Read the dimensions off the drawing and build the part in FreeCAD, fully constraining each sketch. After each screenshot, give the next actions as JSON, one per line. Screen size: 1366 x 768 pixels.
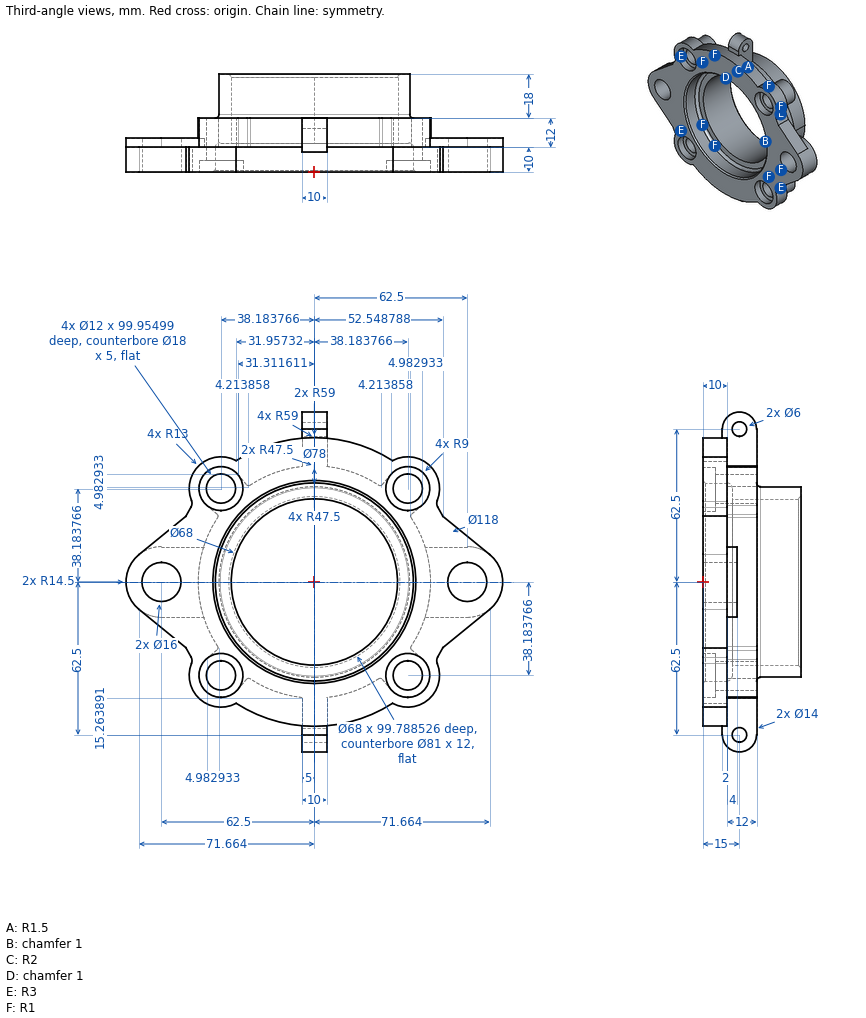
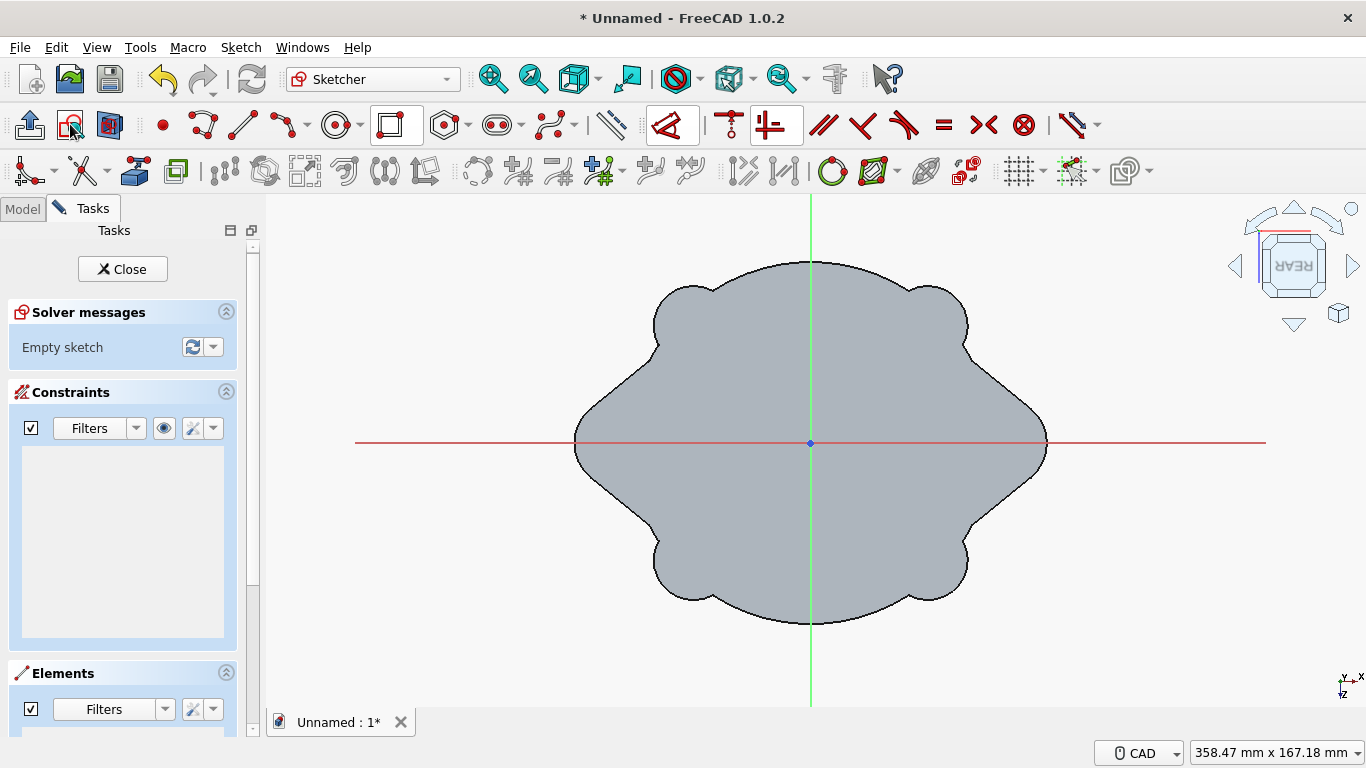
{"action": "left_click", "coordinate": [244, 126]}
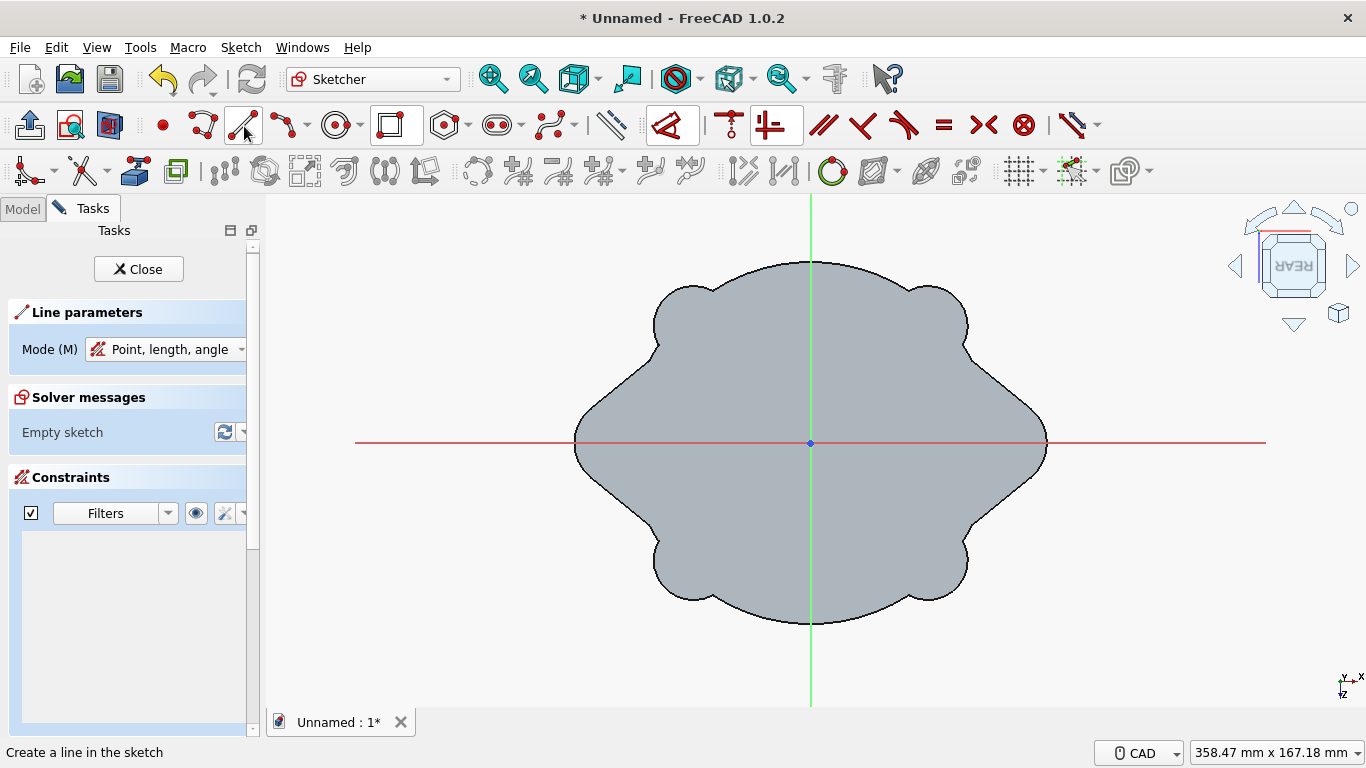
{"action": "left_click", "coordinate": [715, 578]}
{"action": "left_click", "coordinate": [728, 563]}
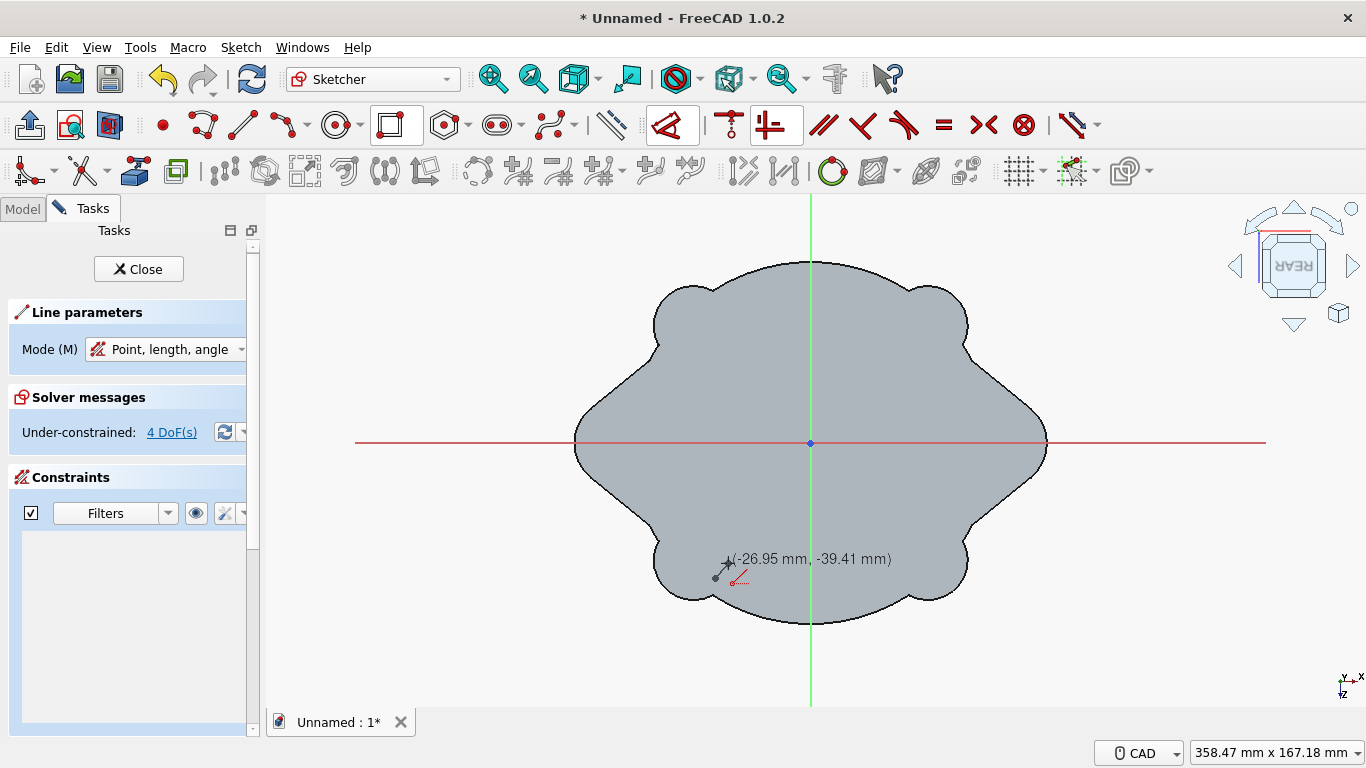
{"action": "left_click", "coordinate": [894, 563]}
{"action": "left_click", "coordinate": [907, 578]}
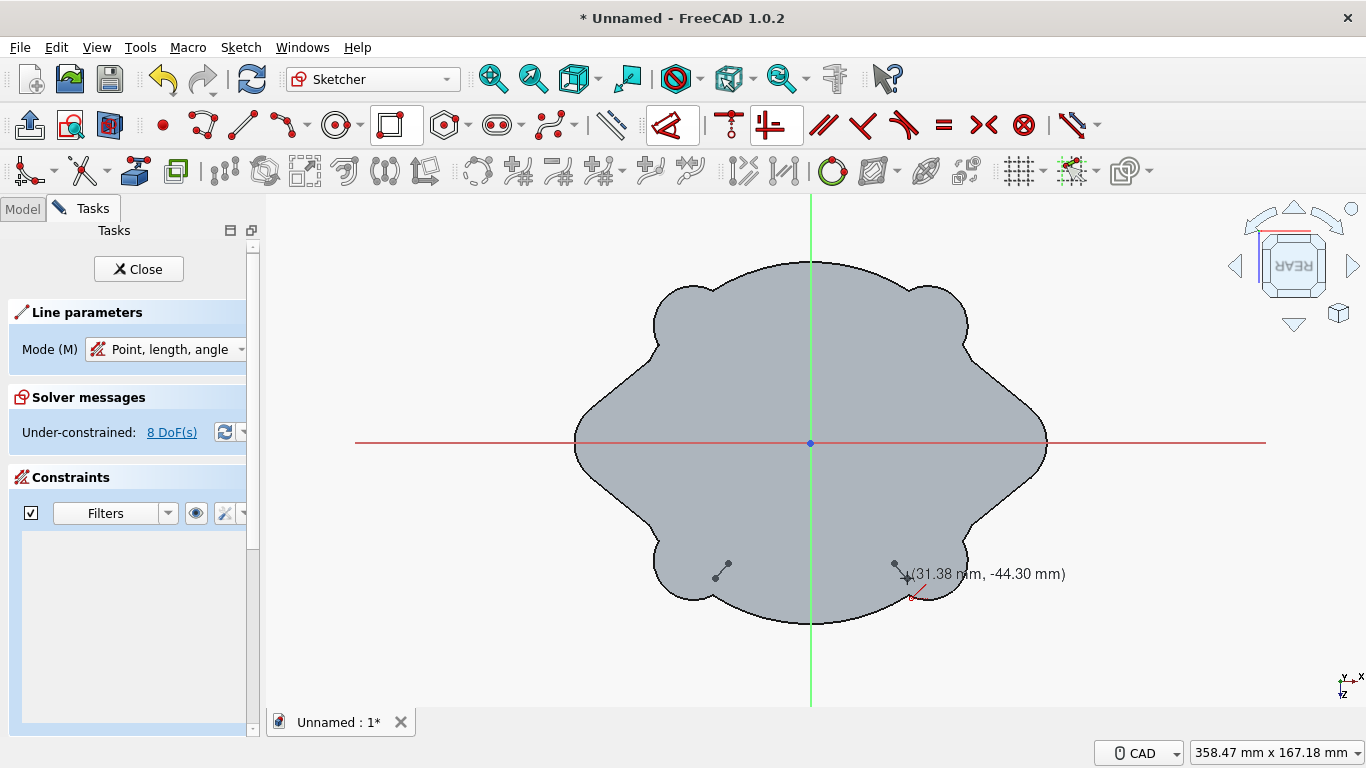
{"action": "left_click", "coordinate": [946, 539]}
{"action": "left_click", "coordinate": [930, 526]}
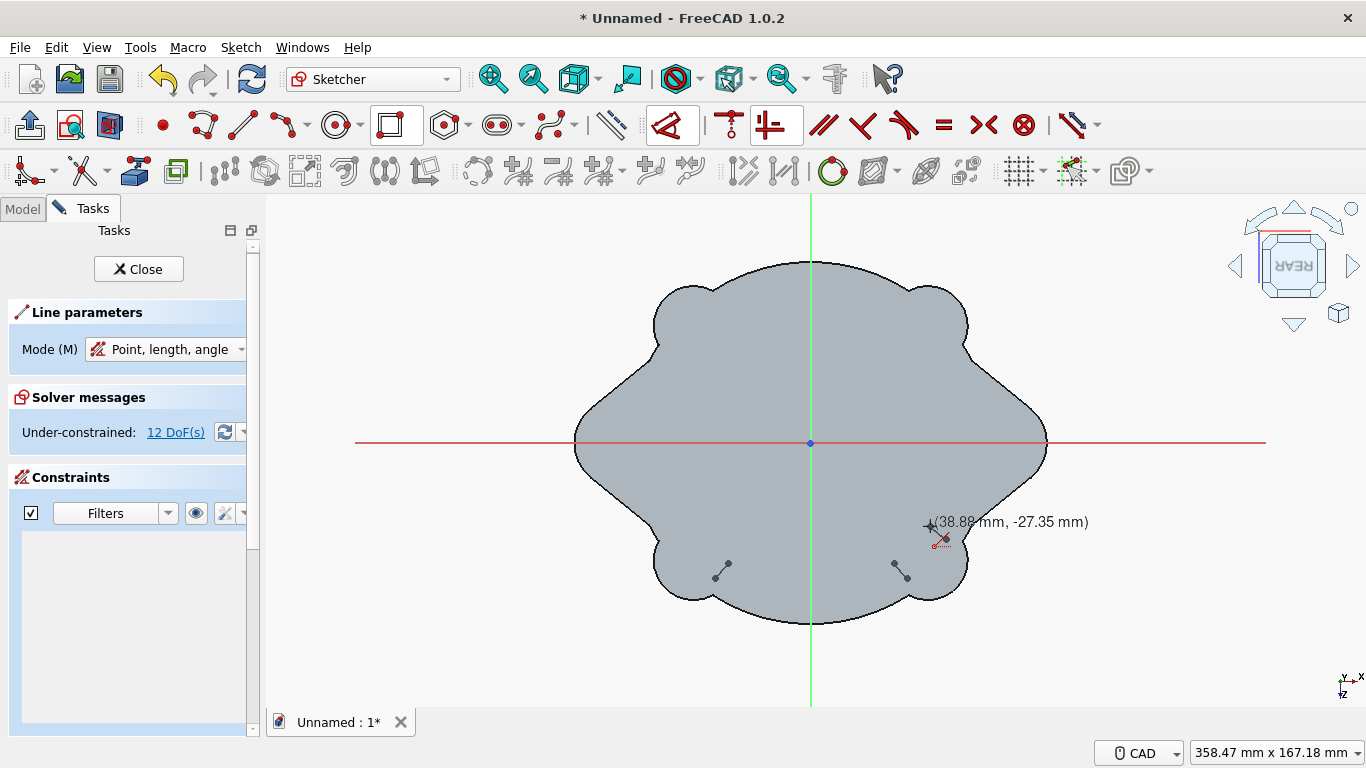
{"action": "left_click", "coordinate": [930, 360]}
{"action": "left_click", "coordinate": [946, 347]}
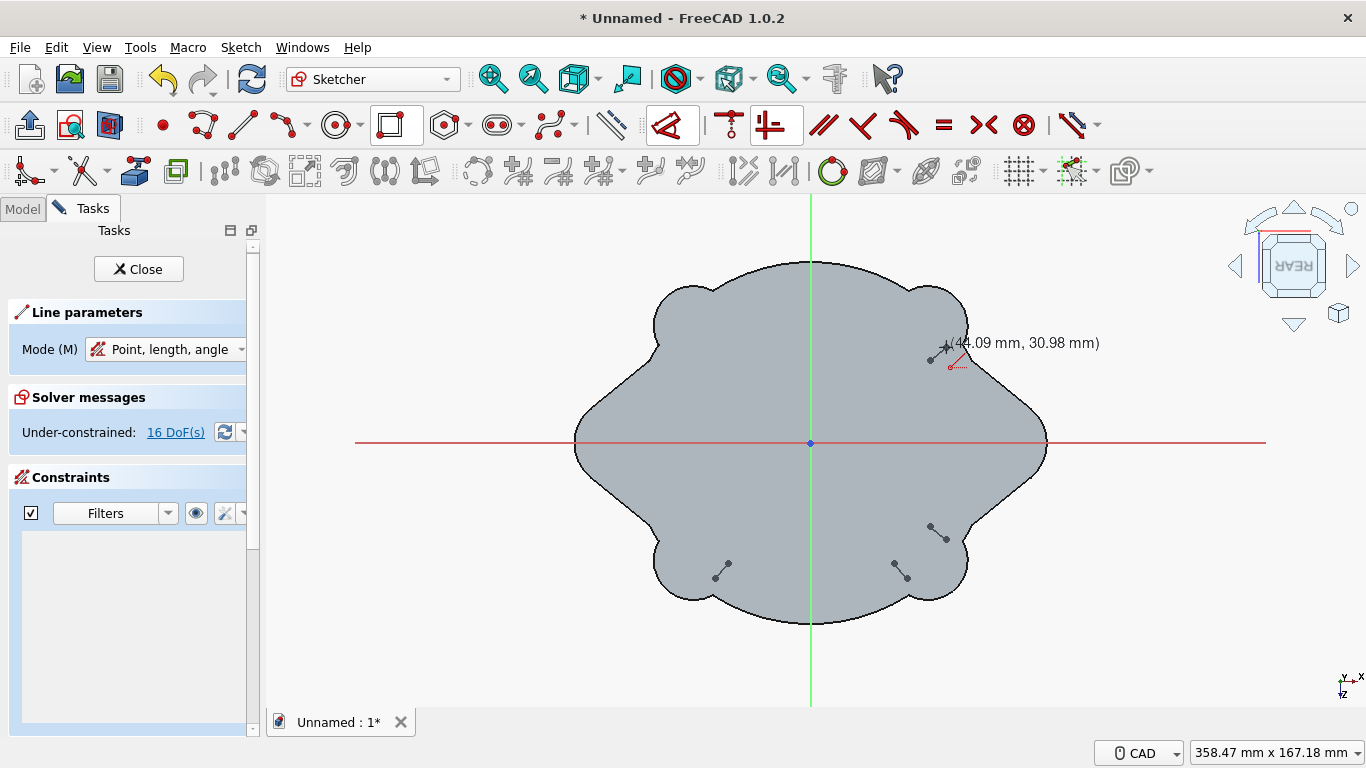
{"action": "left_click", "coordinate": [907, 308]}
{"action": "left_click", "coordinate": [894, 323]}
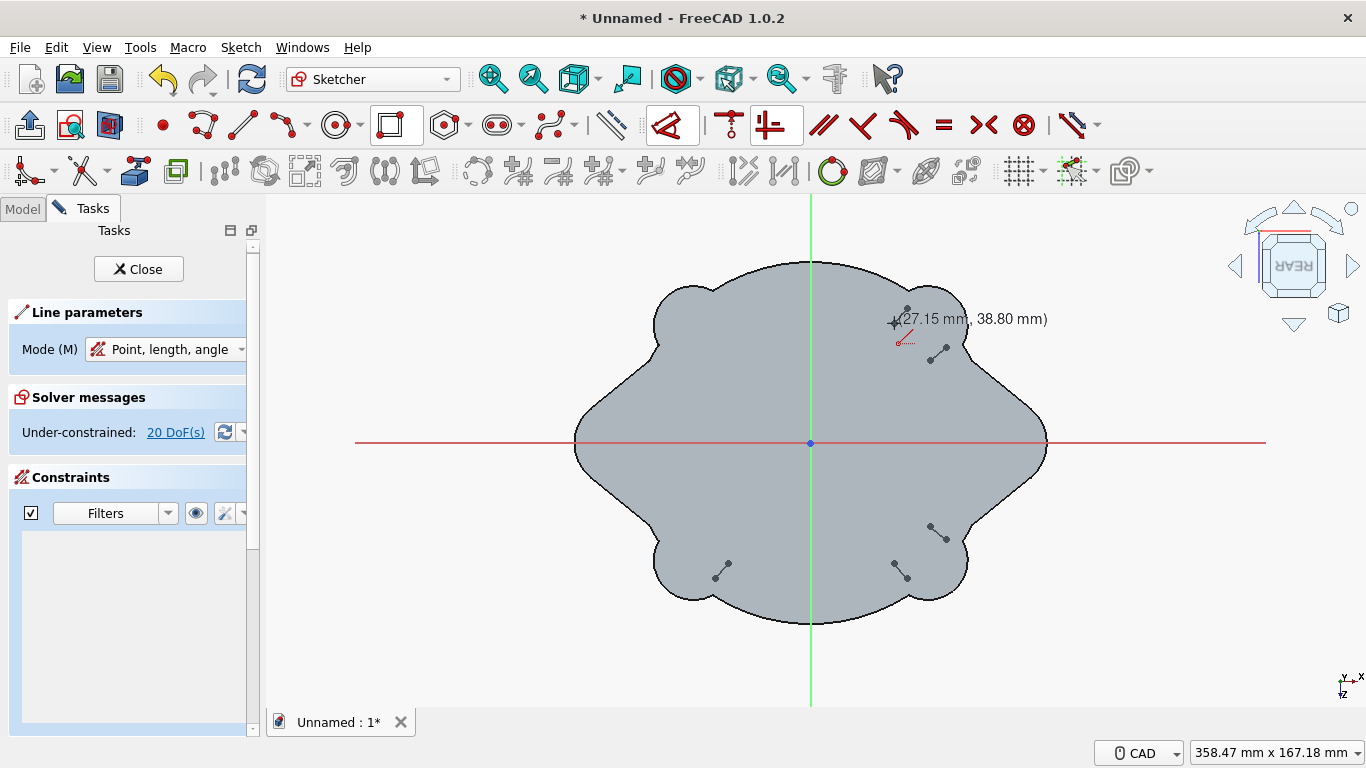
{"action": "left_click", "coordinate": [728, 323]}
{"action": "left_click", "coordinate": [715, 308]}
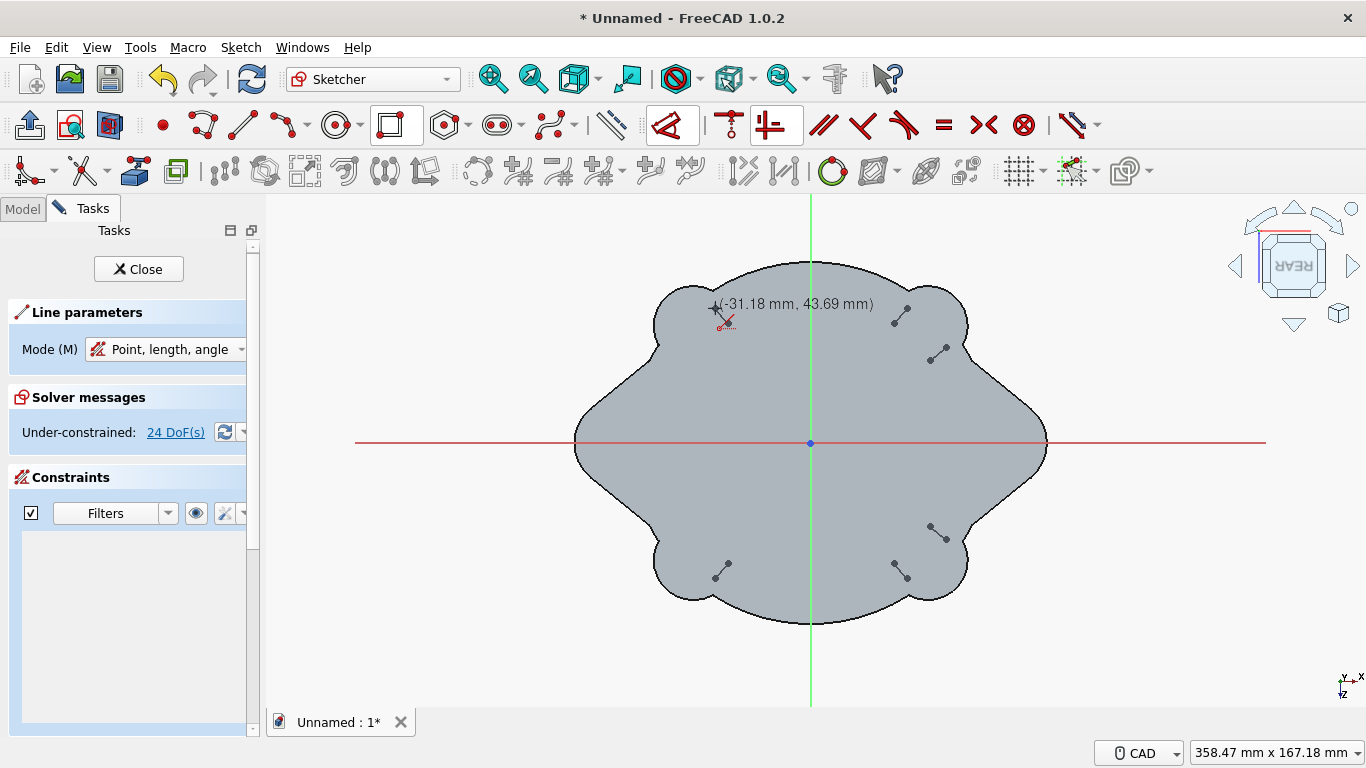
{"action": "left_click", "coordinate": [676, 347]}
{"action": "left_click", "coordinate": [691, 360]}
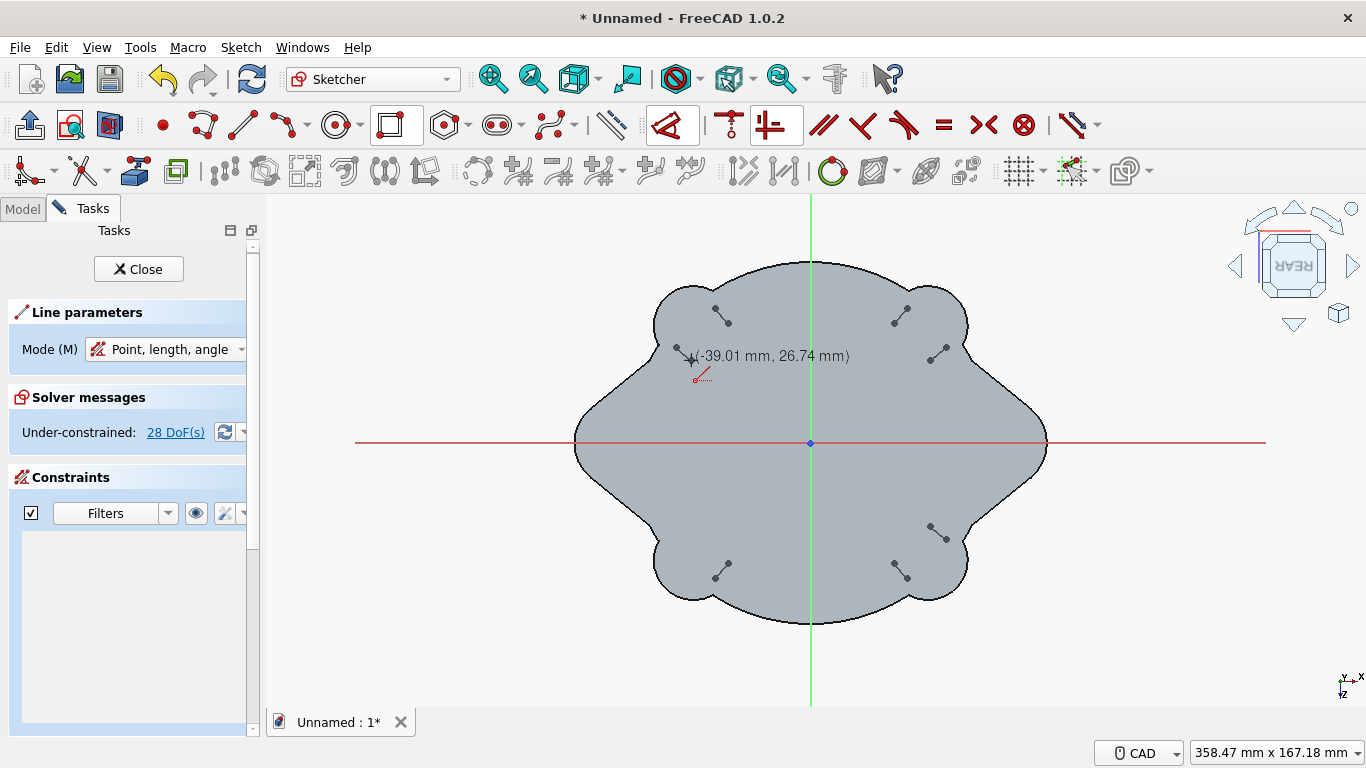
{"action": "left_click", "coordinate": [691, 526]}
{"action": "left_click", "coordinate": [676, 539]}